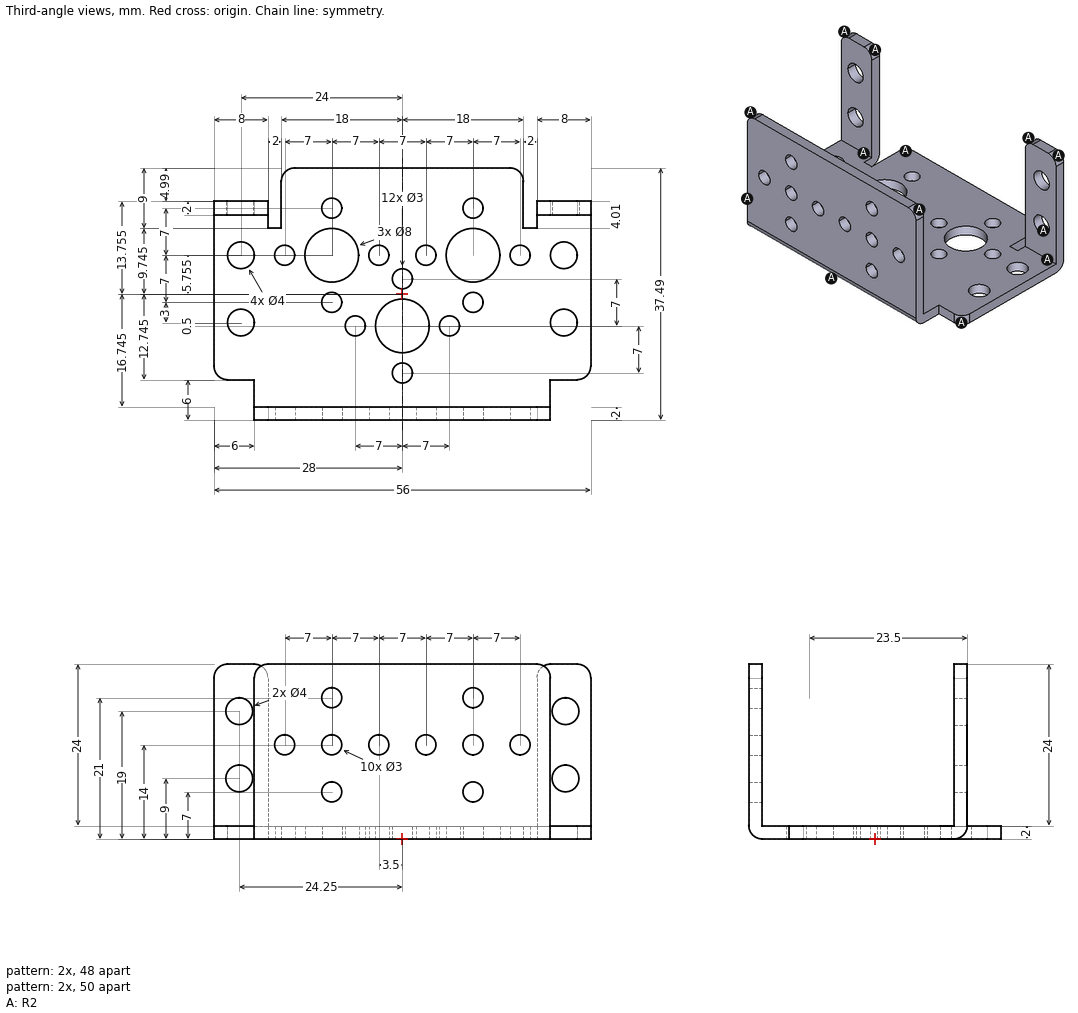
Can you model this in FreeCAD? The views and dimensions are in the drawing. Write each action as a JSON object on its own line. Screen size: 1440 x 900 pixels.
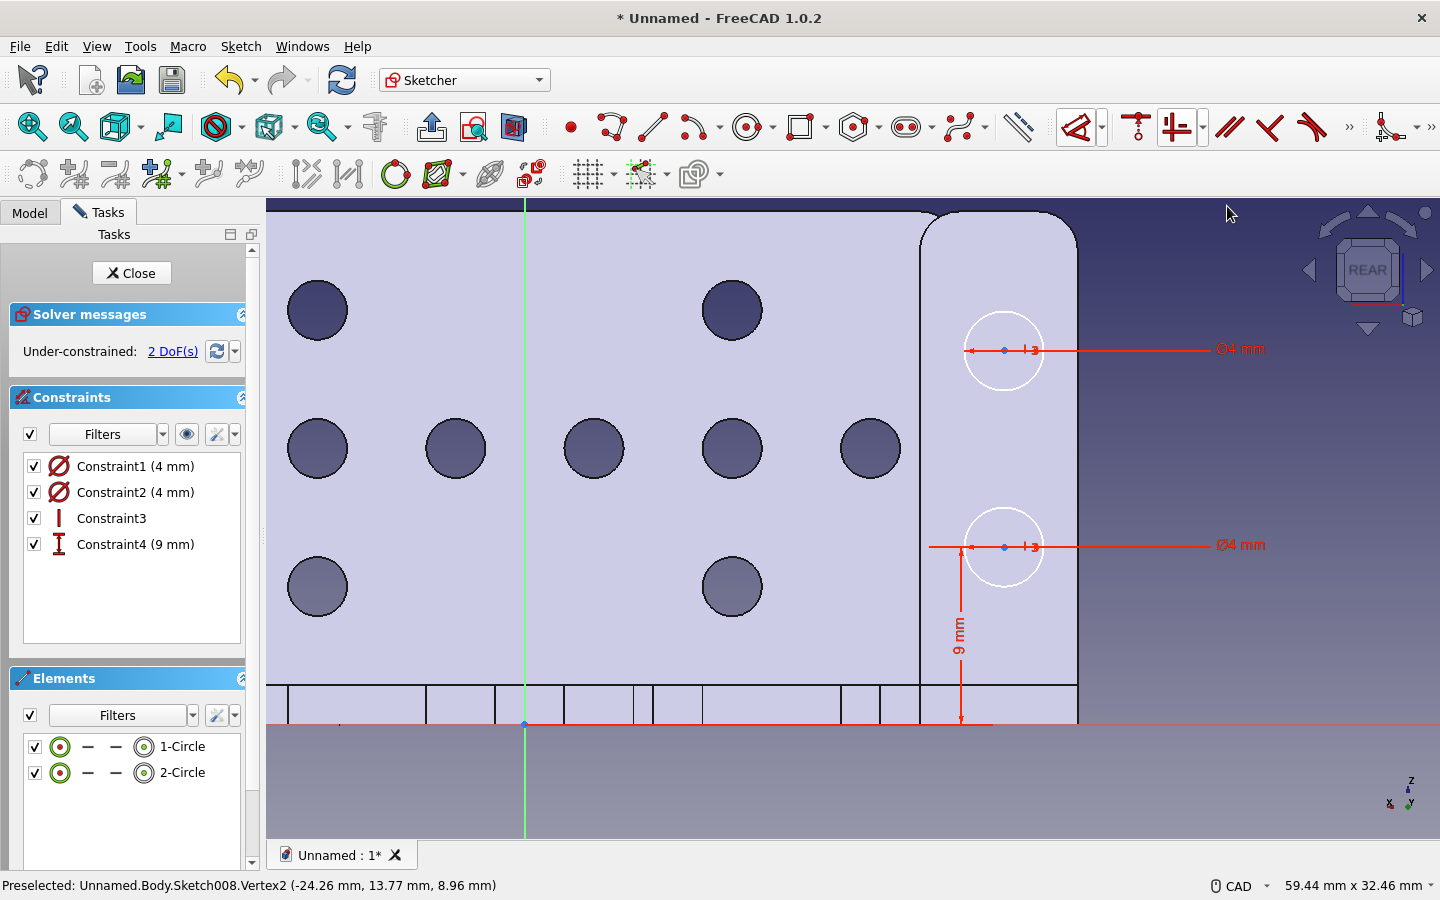
{"action": "left_click", "coordinate": [1004, 351]}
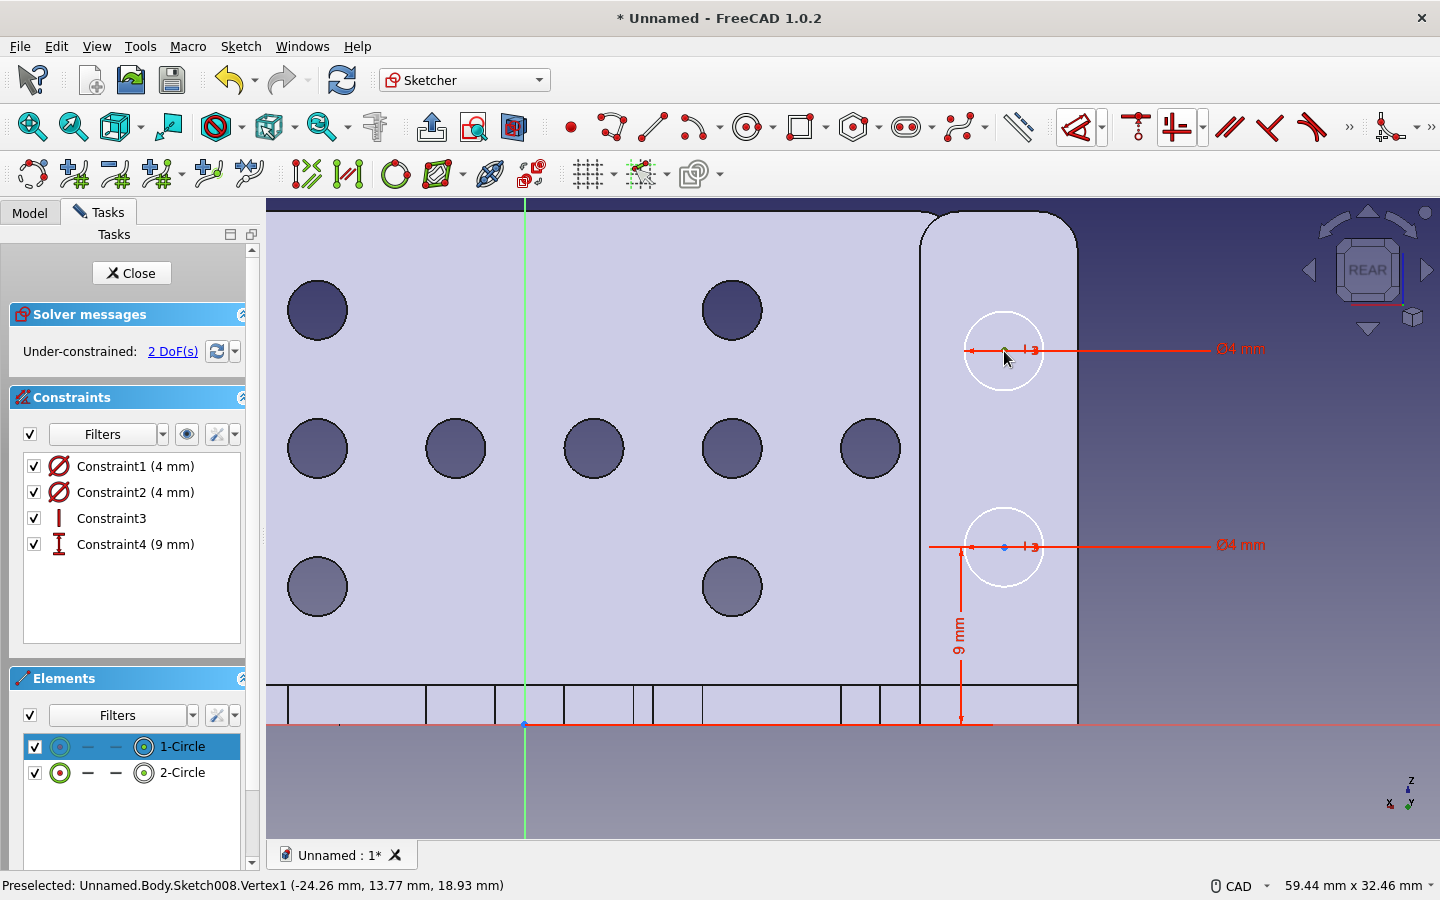
{"action": "key", "text": "i"}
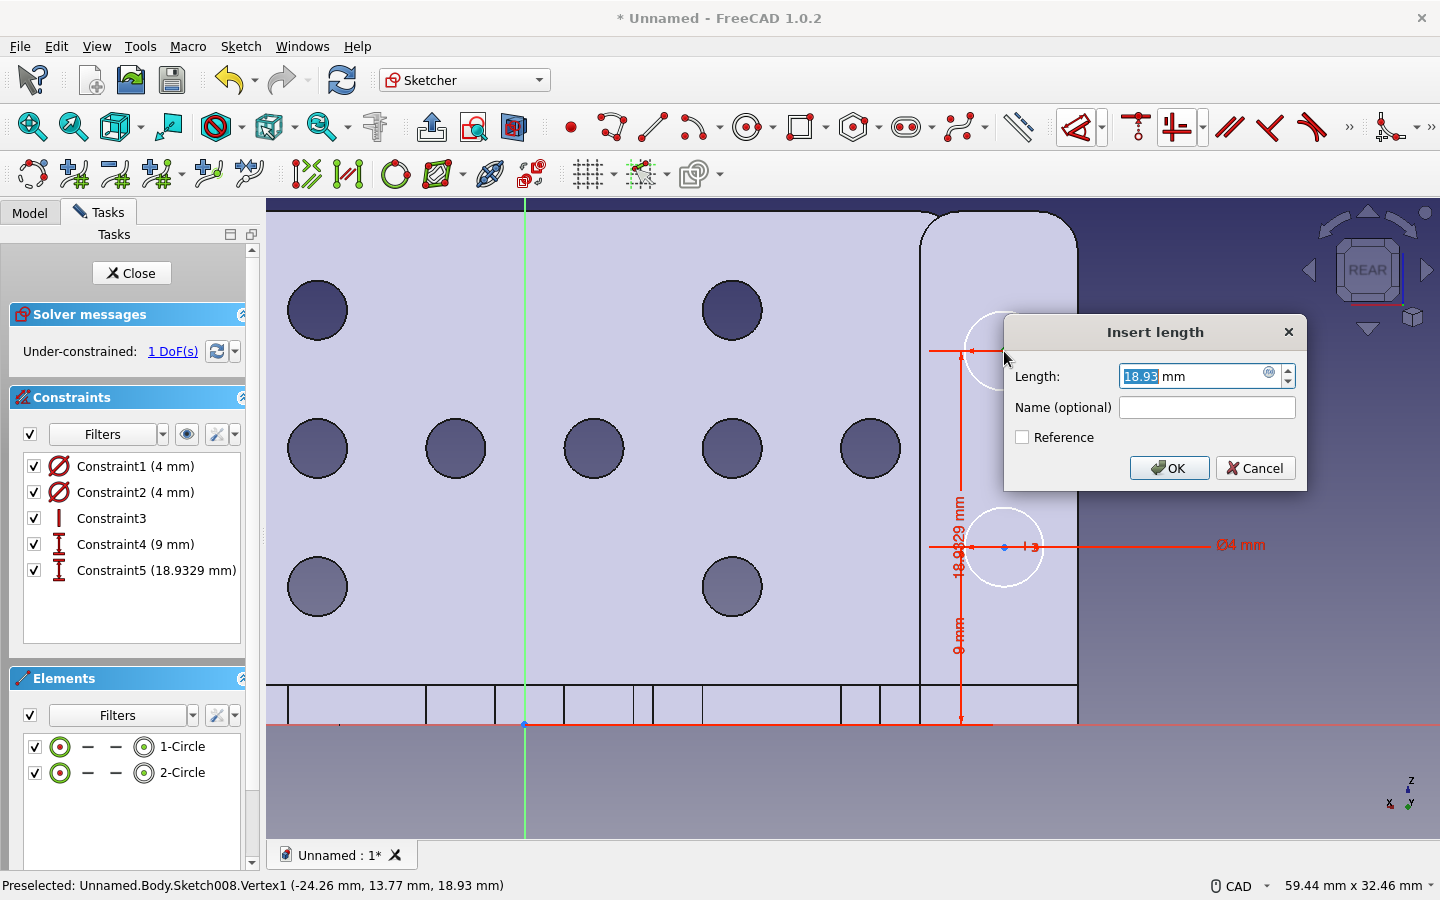
{"action": "type", "text": "19"}
{"action": "key", "text": "Return"}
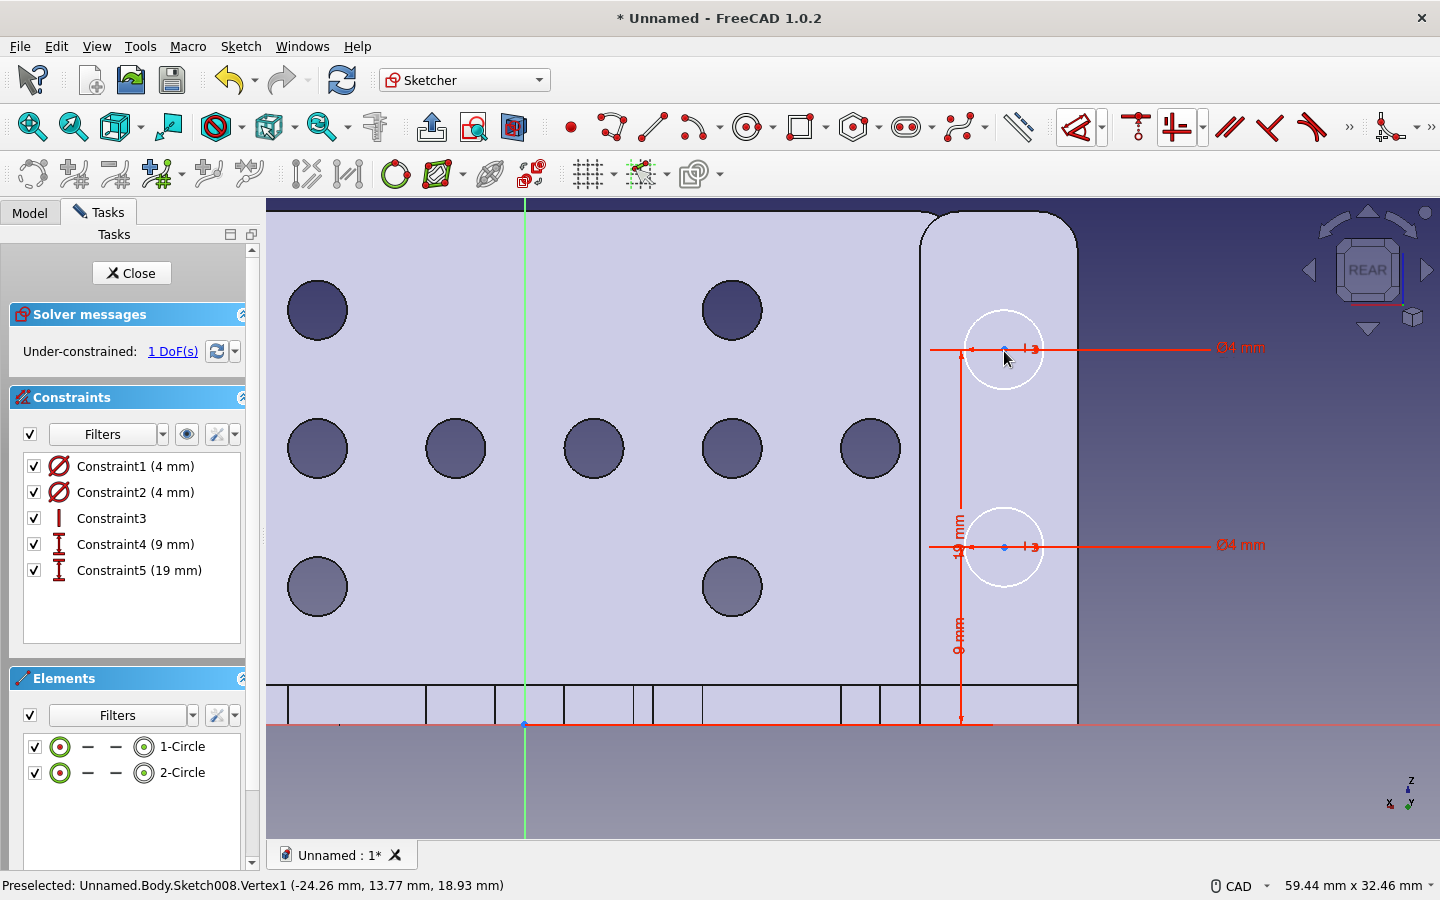
{"action": "left_click", "coordinate": [1004, 350]}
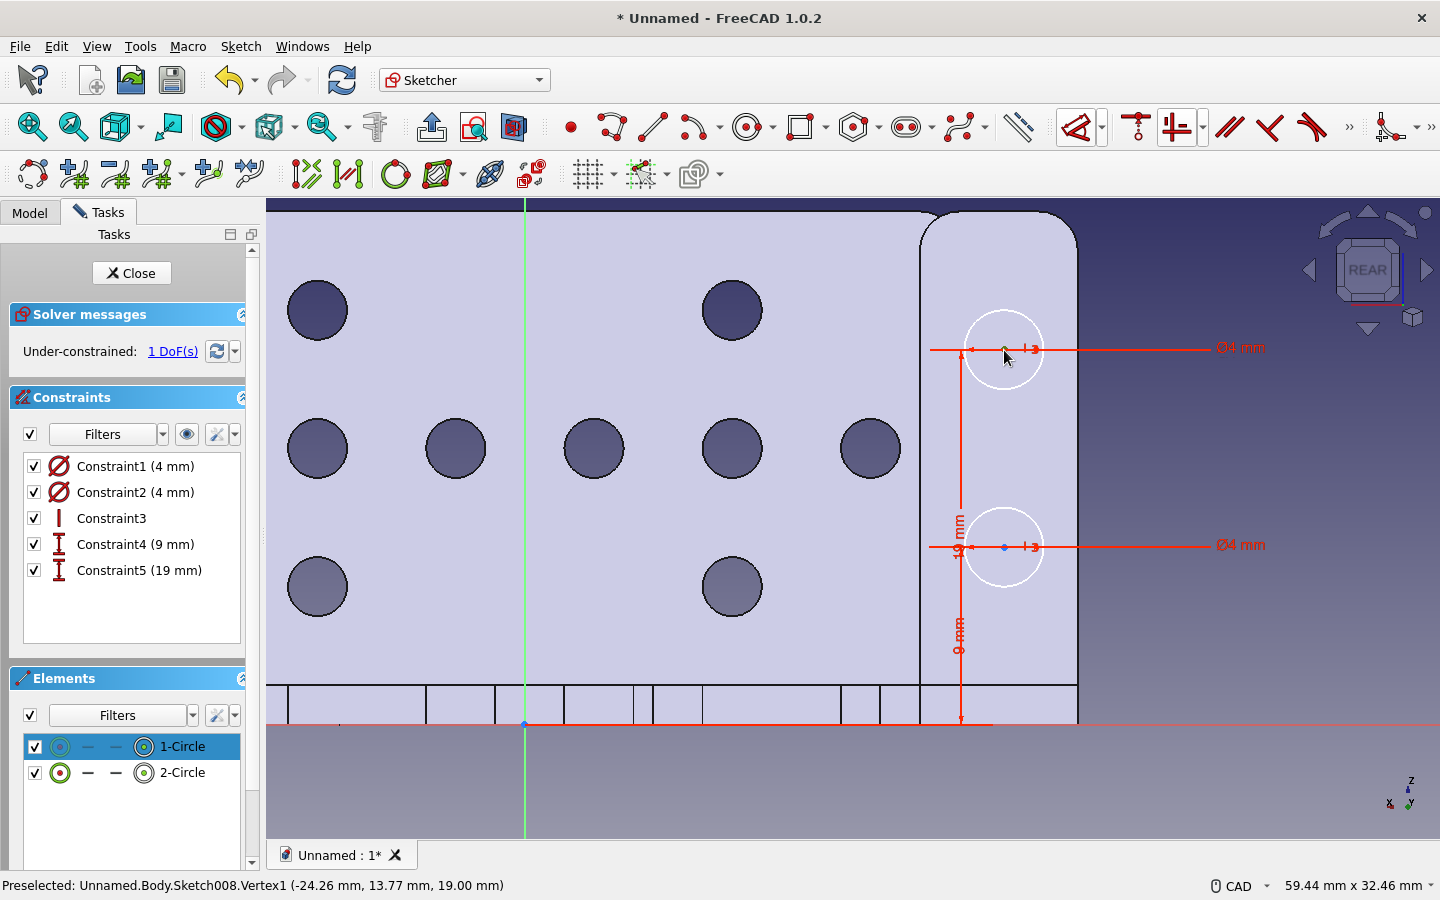
{"action": "key", "text": "l"}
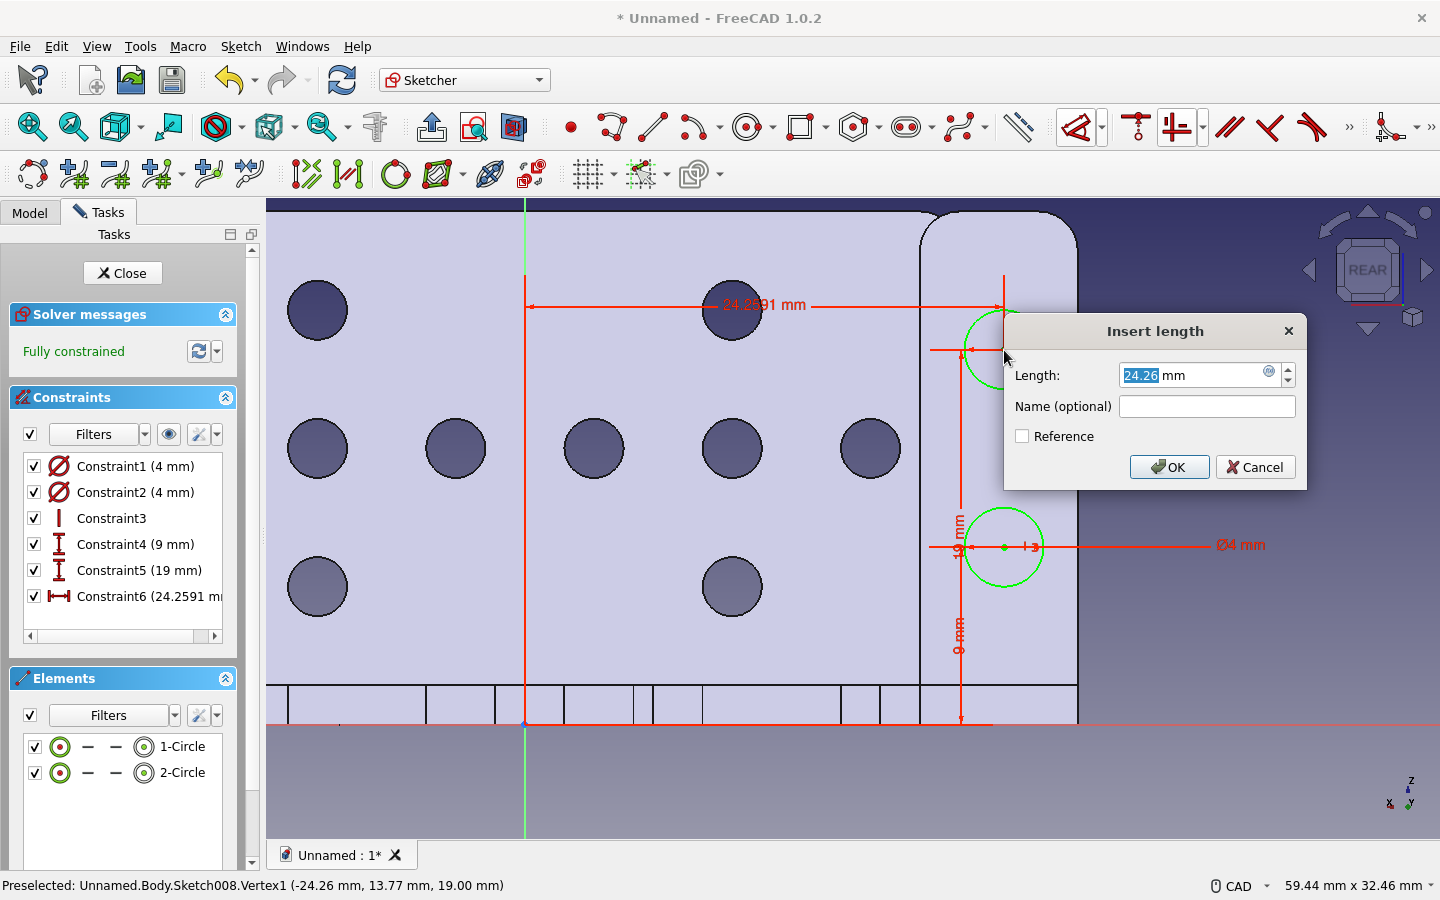
{"action": "type", "text": "24.25"}
{"action": "key", "text": "Return"}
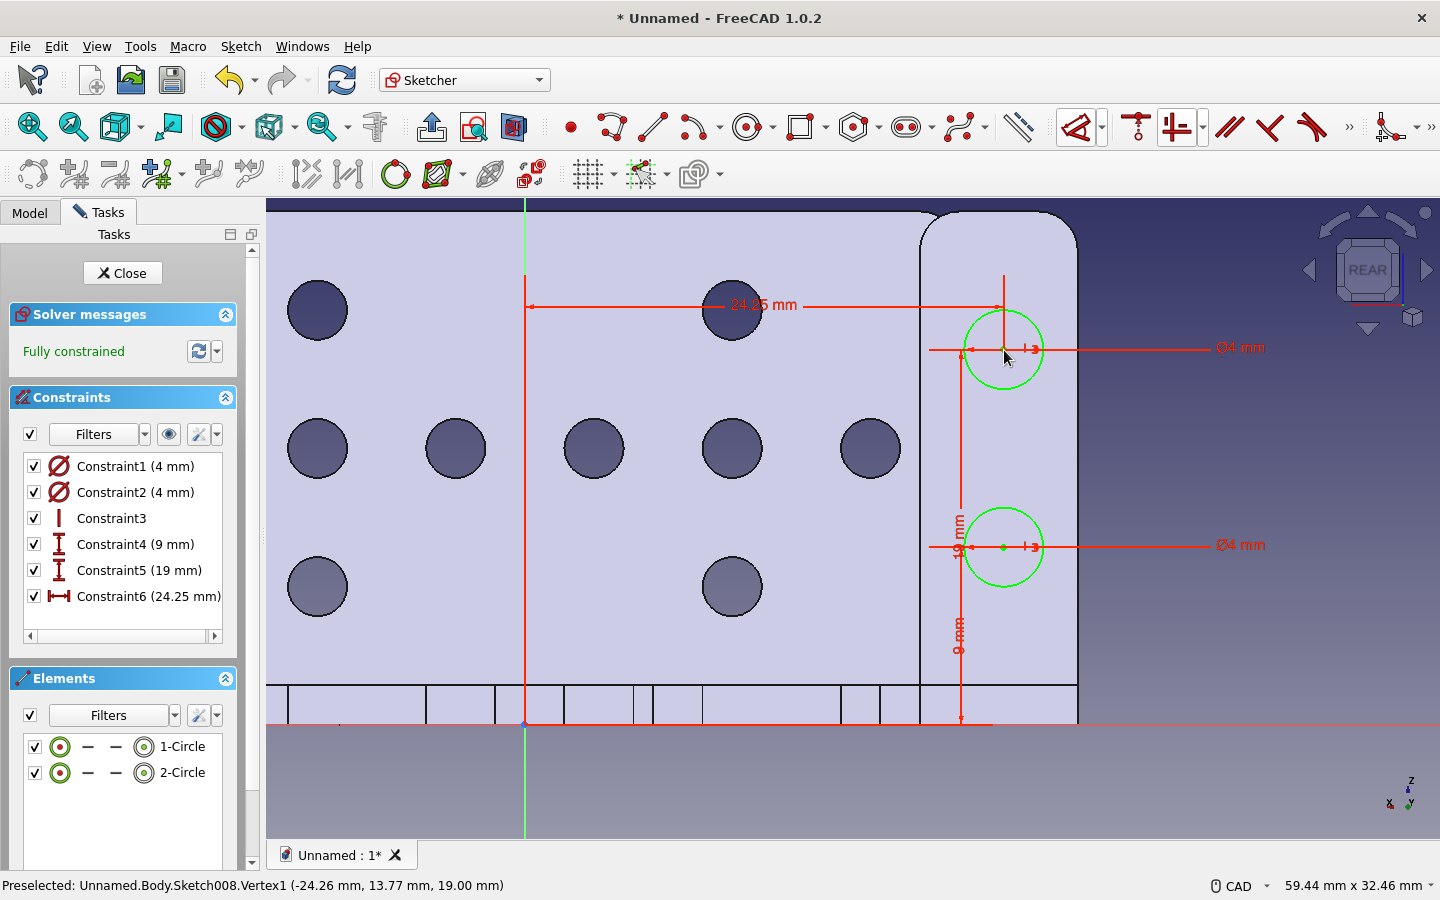
{"action": "left_click", "coordinate": [123, 273]}